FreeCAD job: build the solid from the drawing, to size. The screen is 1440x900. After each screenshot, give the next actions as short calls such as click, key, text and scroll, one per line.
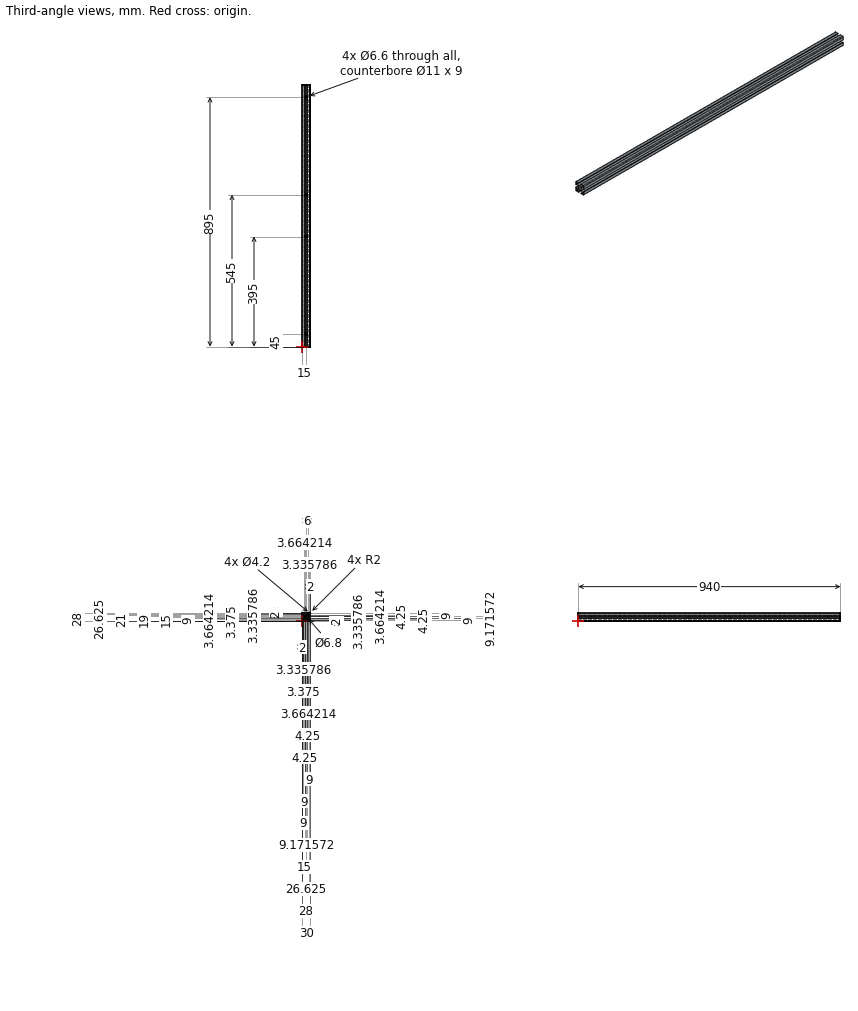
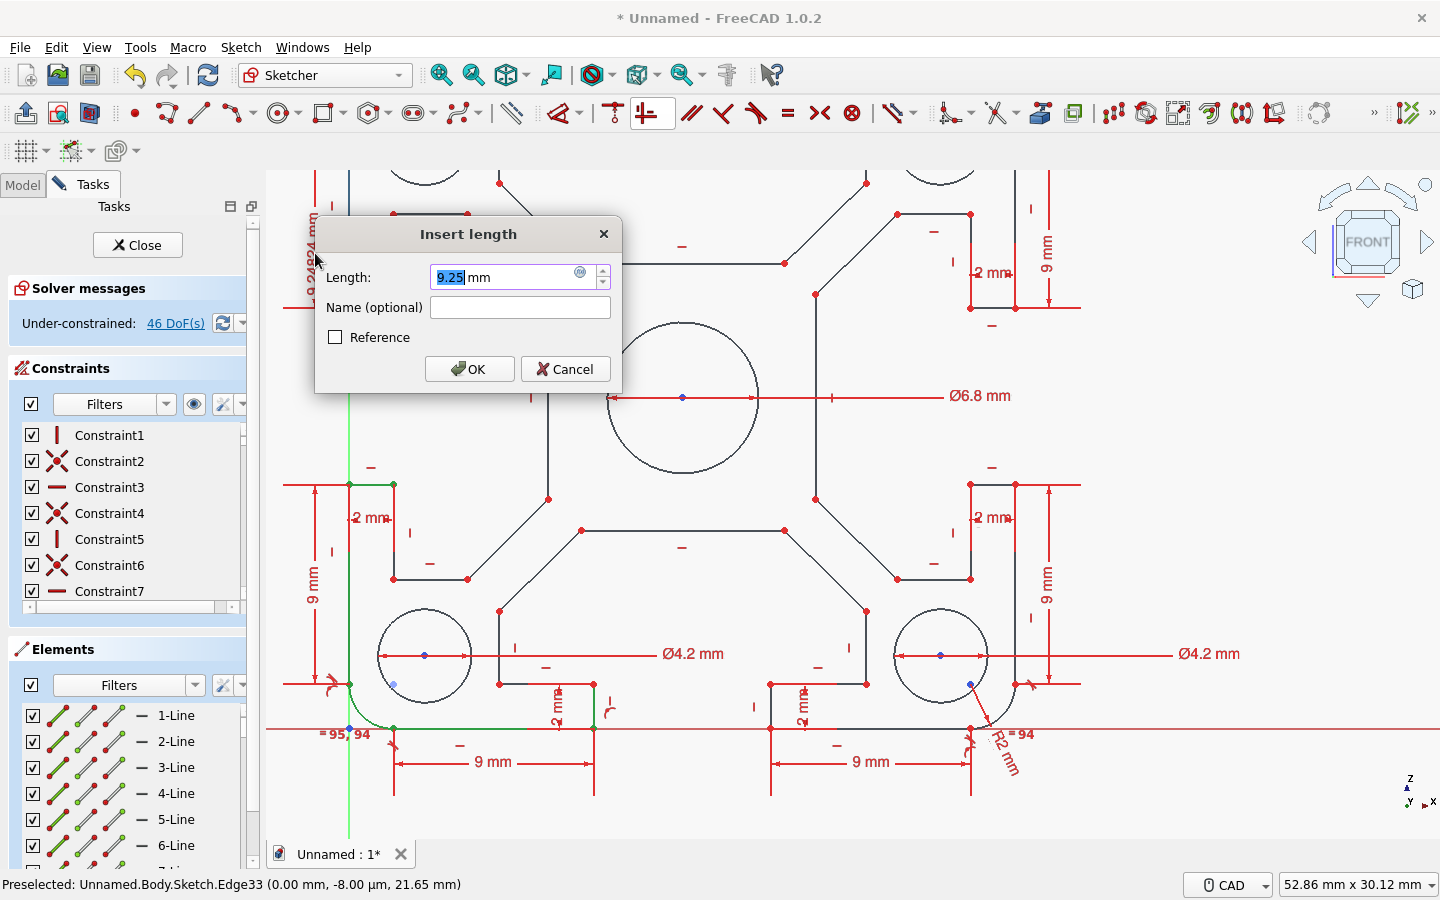
text(9)
key(Return)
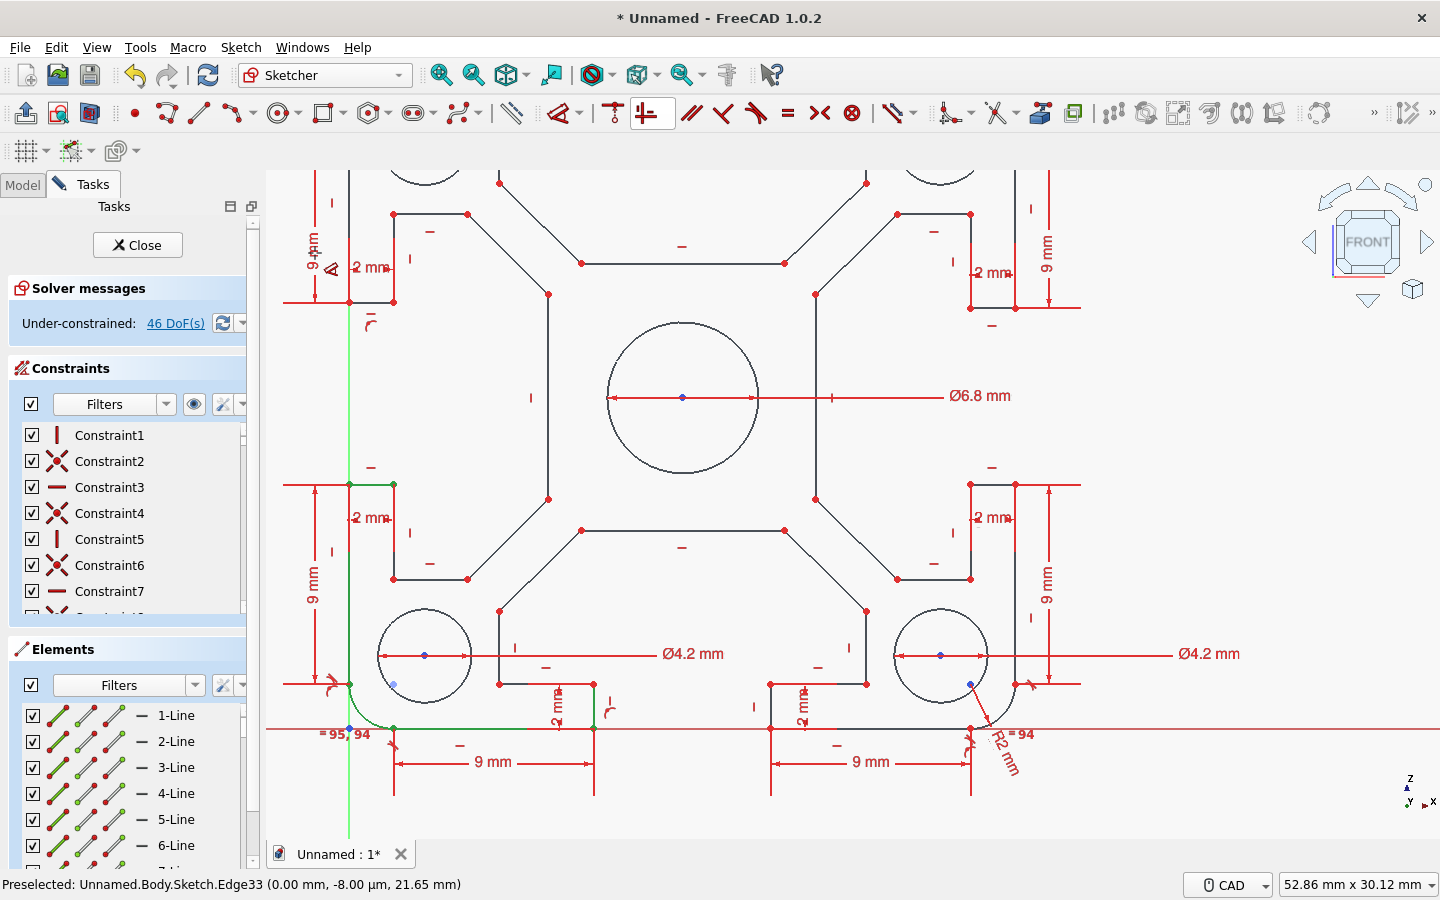
scroll(992, 726, down, 2)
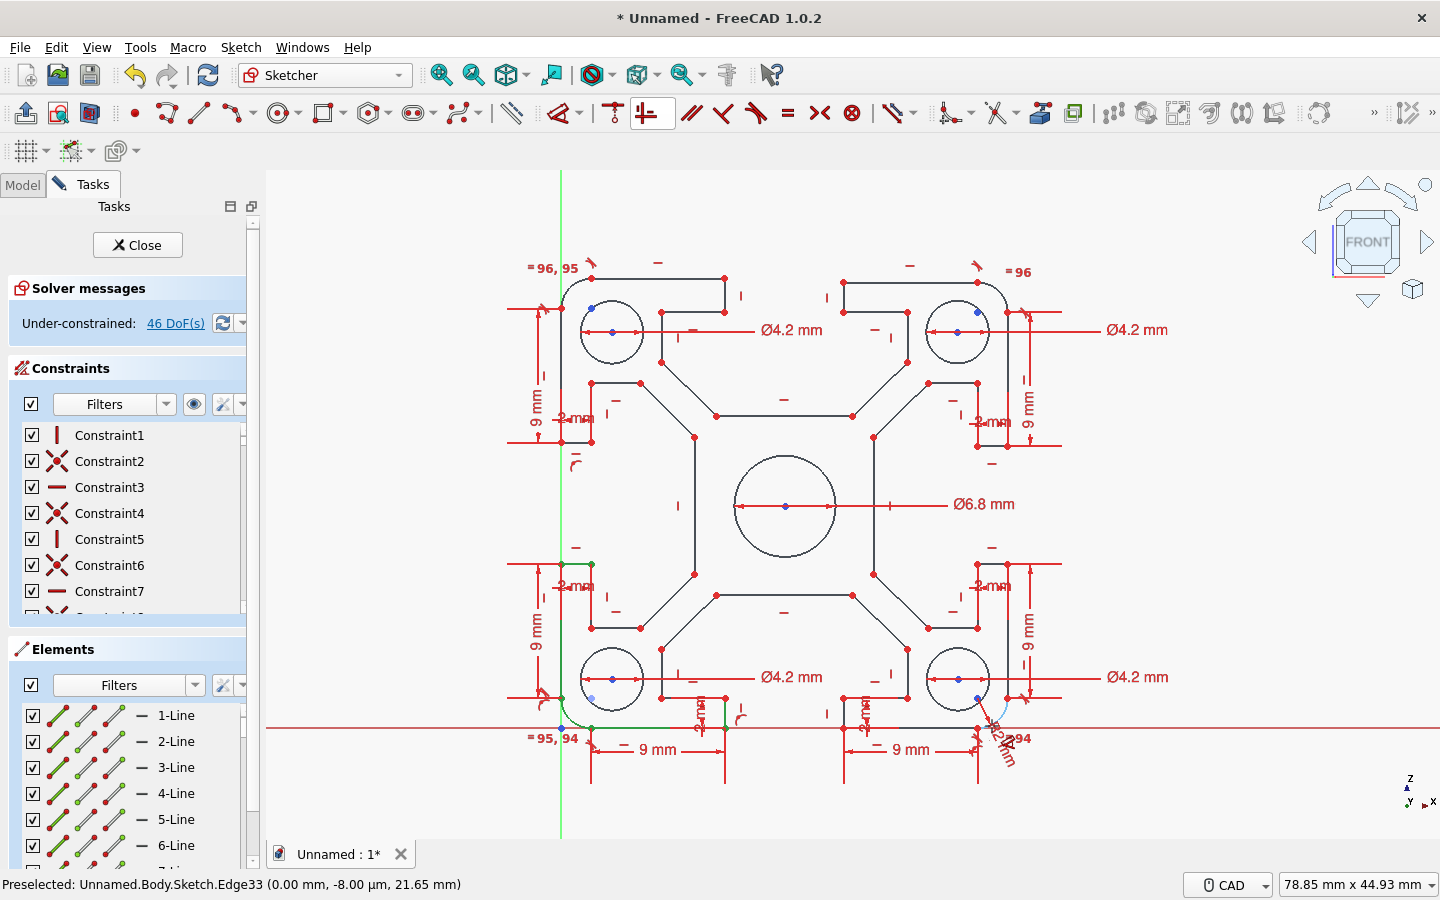
click(631, 279)
click(658, 245)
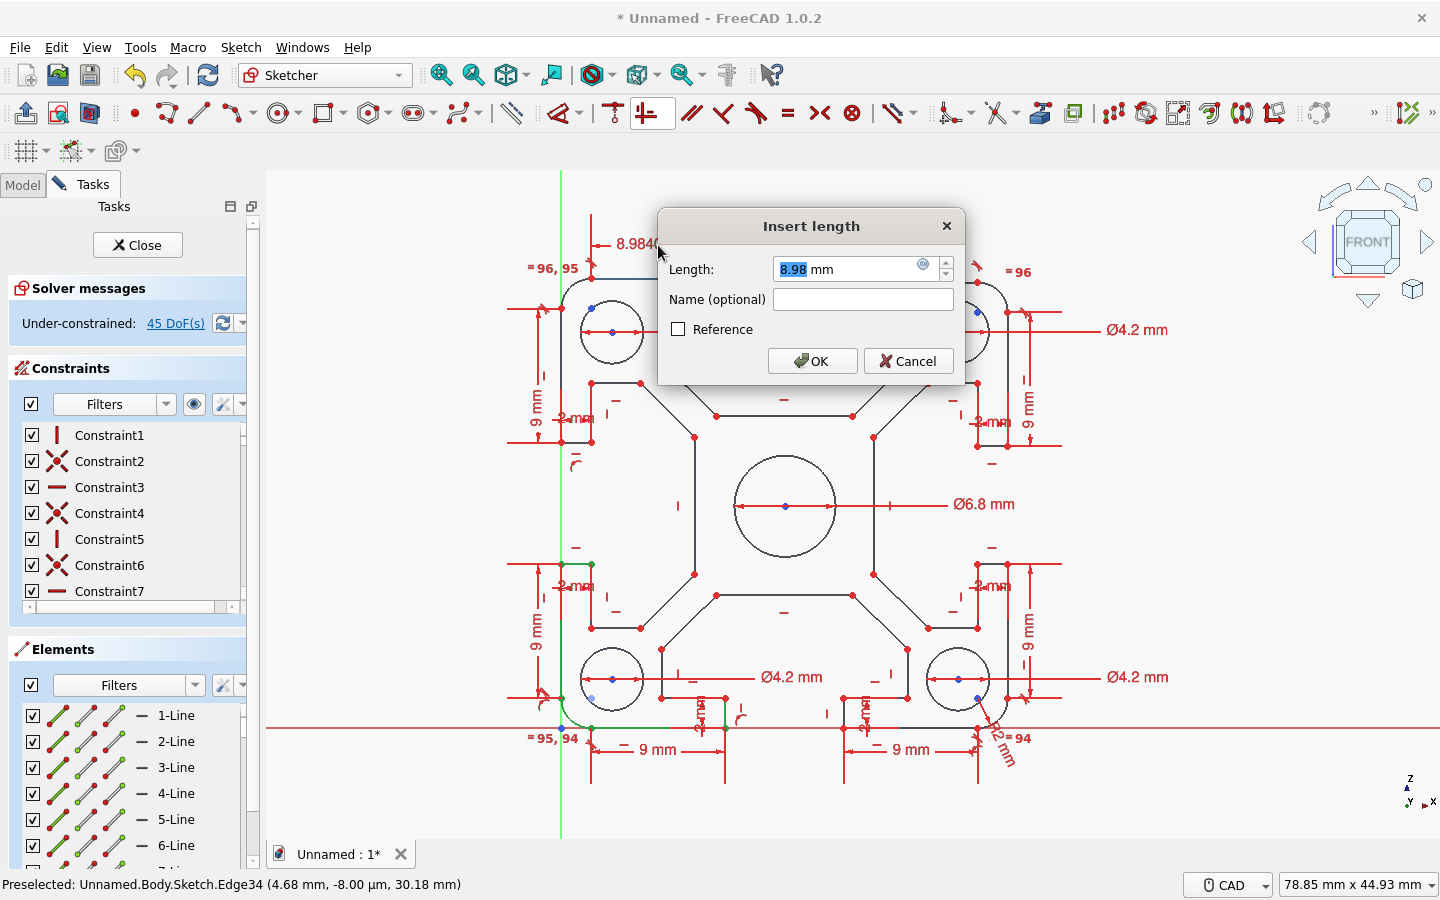
text(9)
key(Return)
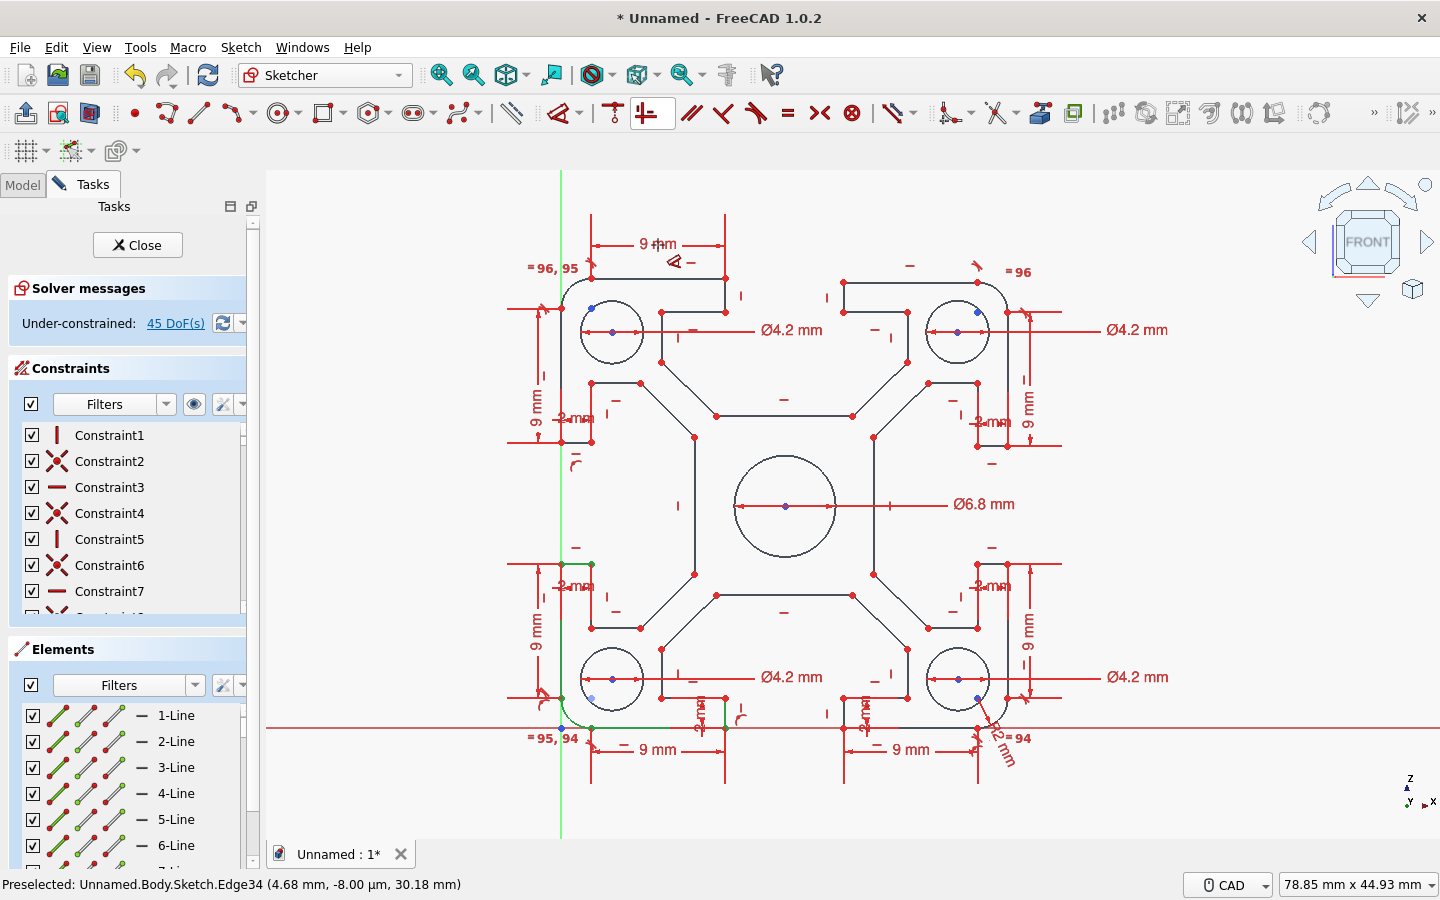
scroll(725, 289, up, 2)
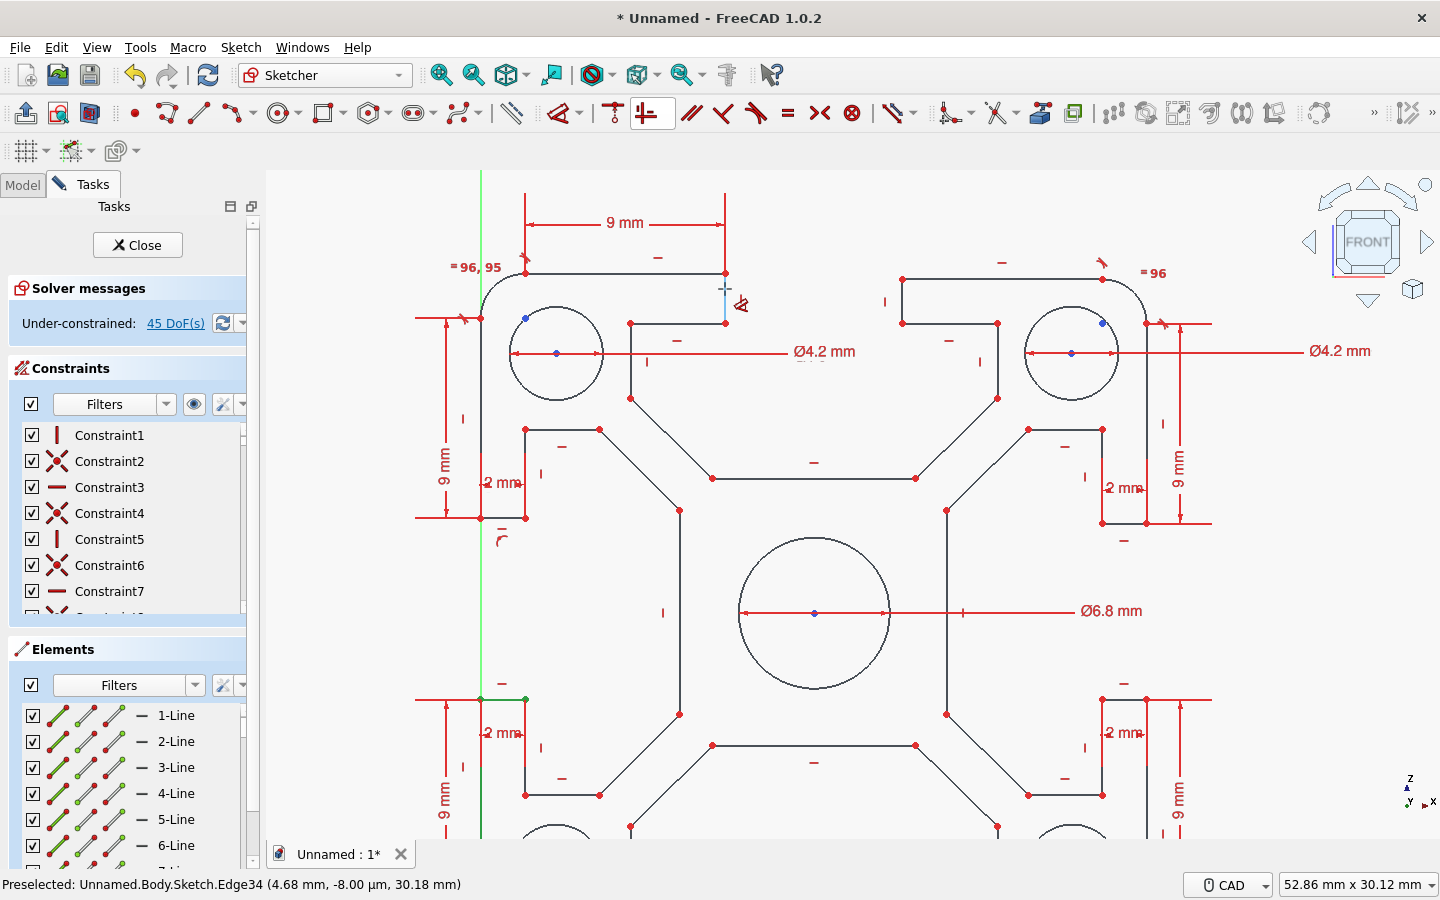
click(725, 289)
click(691, 299)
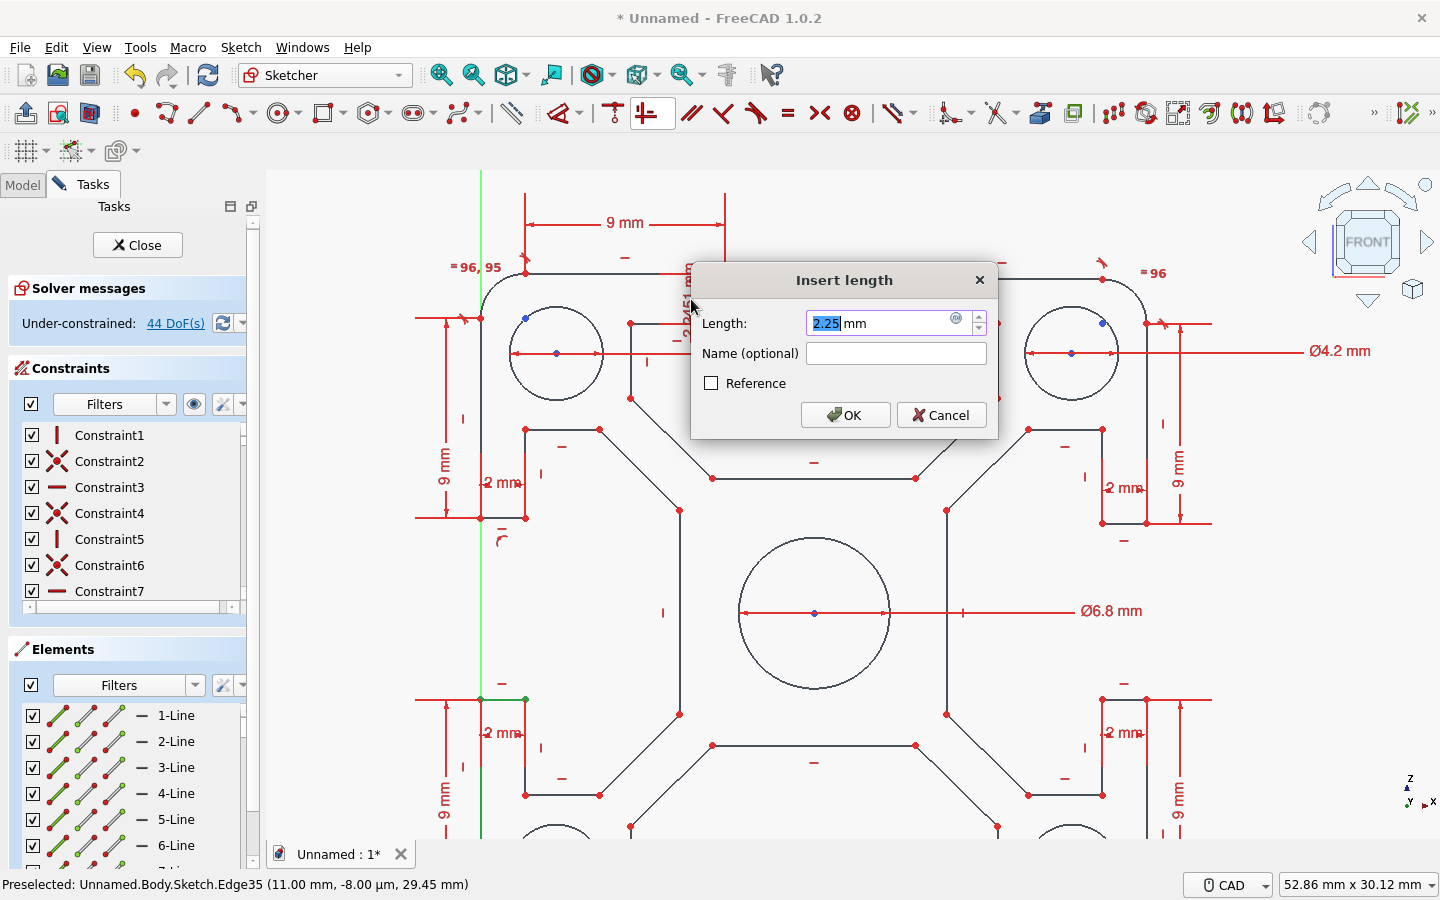
text(2)
key(Return)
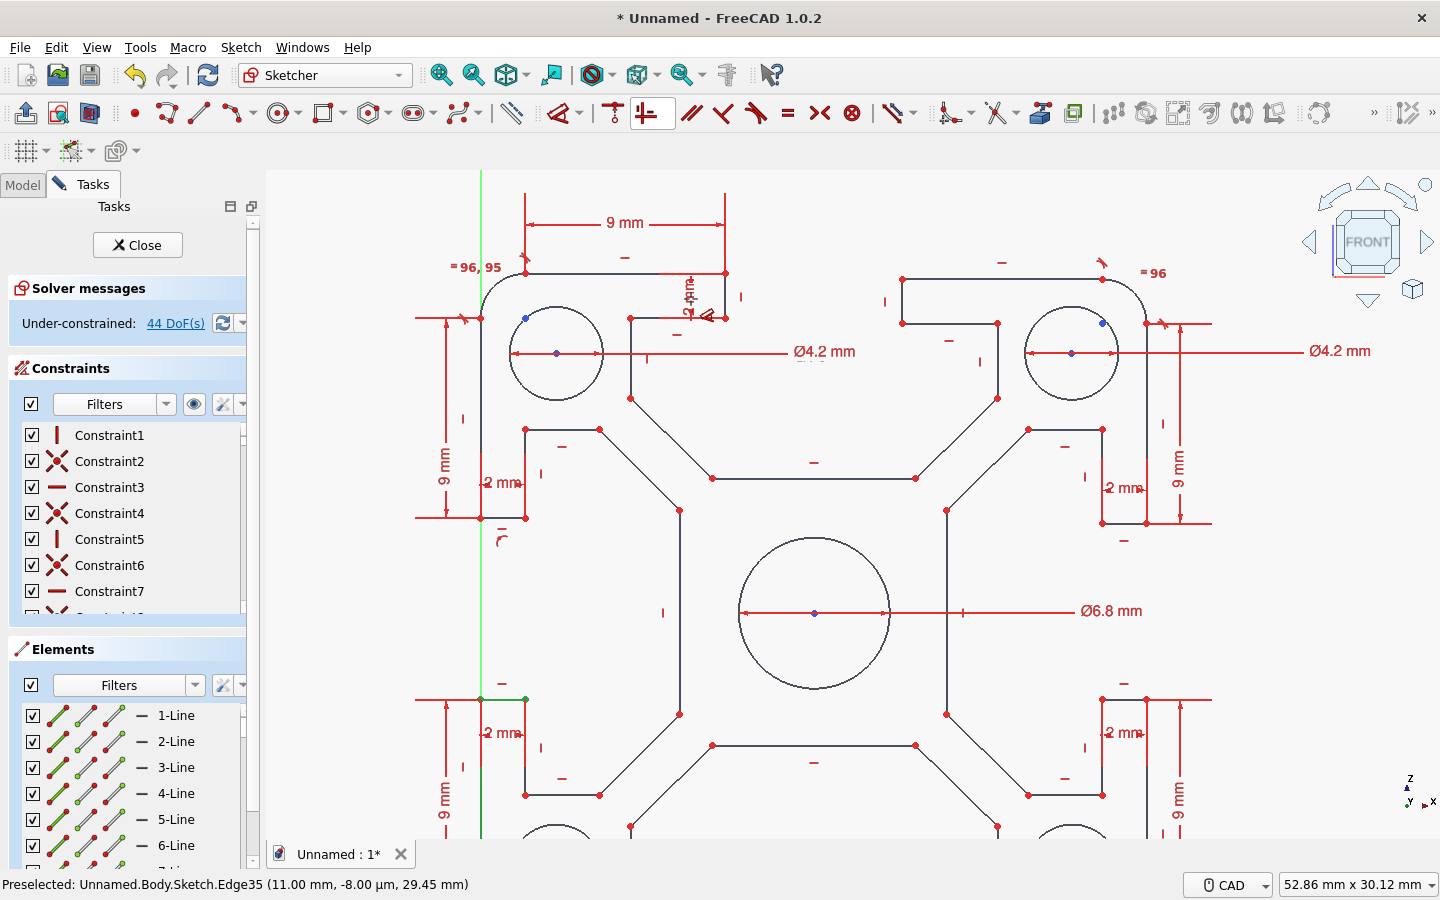
click(902, 310)
click(936, 302)